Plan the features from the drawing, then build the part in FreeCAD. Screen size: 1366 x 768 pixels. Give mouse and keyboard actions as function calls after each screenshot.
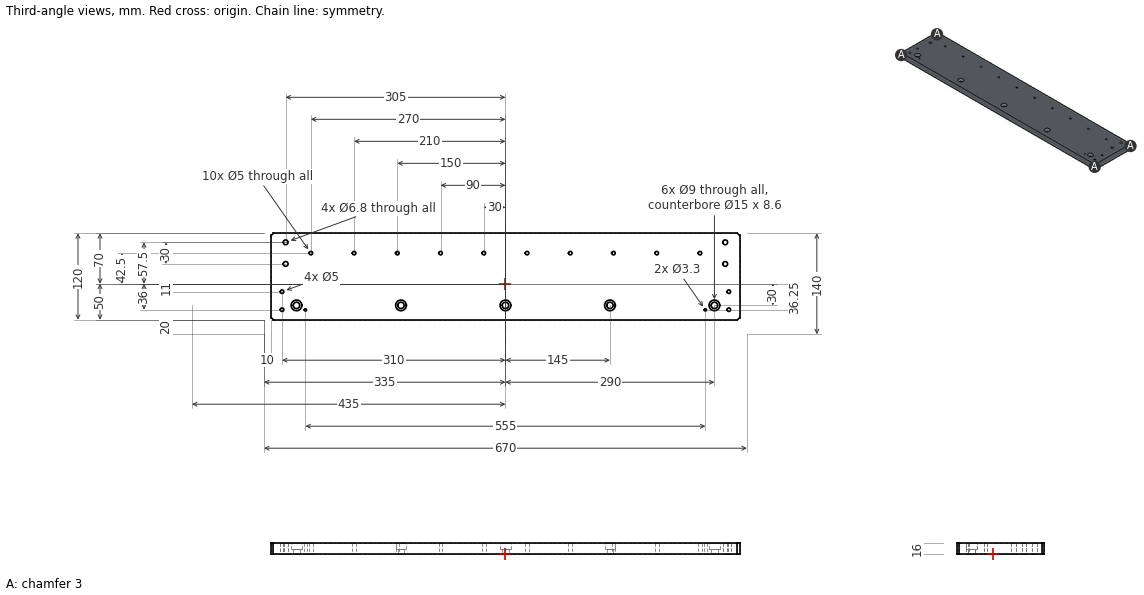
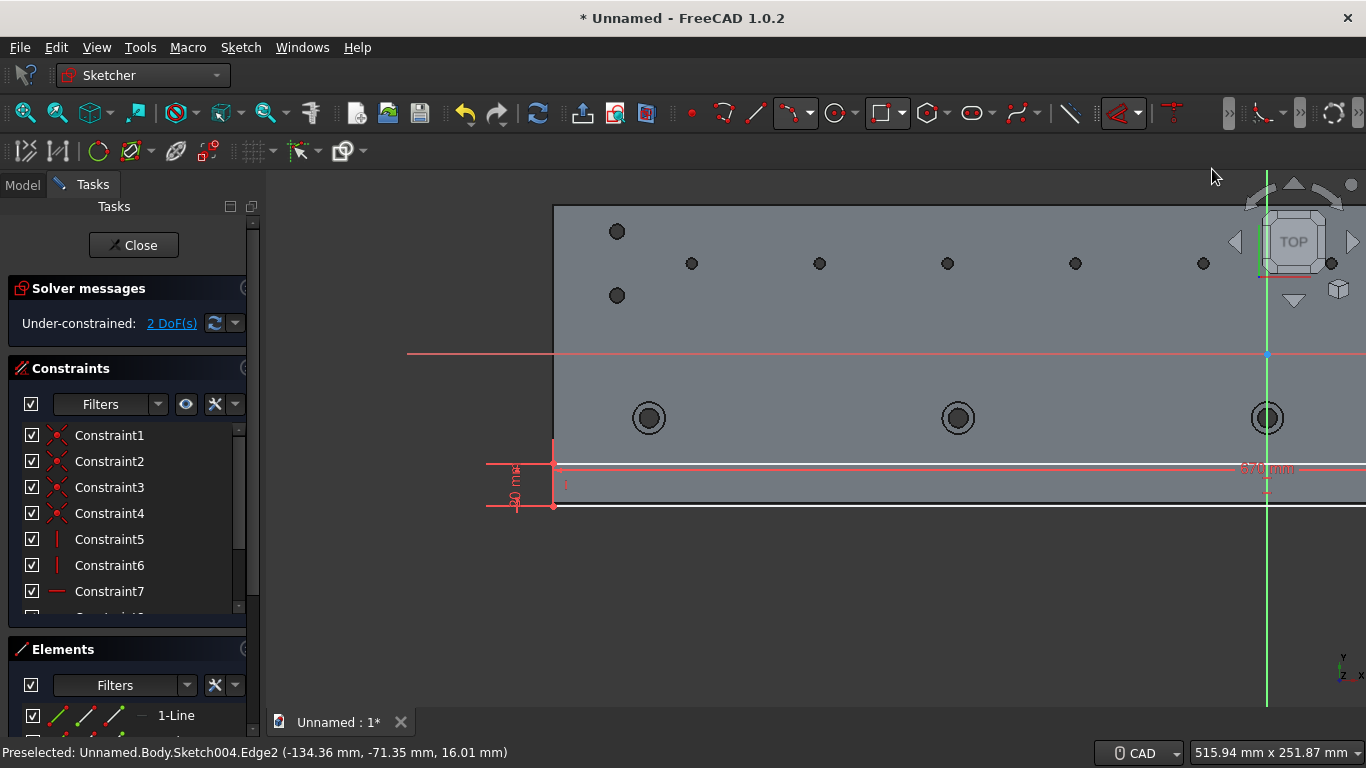
click(553, 464)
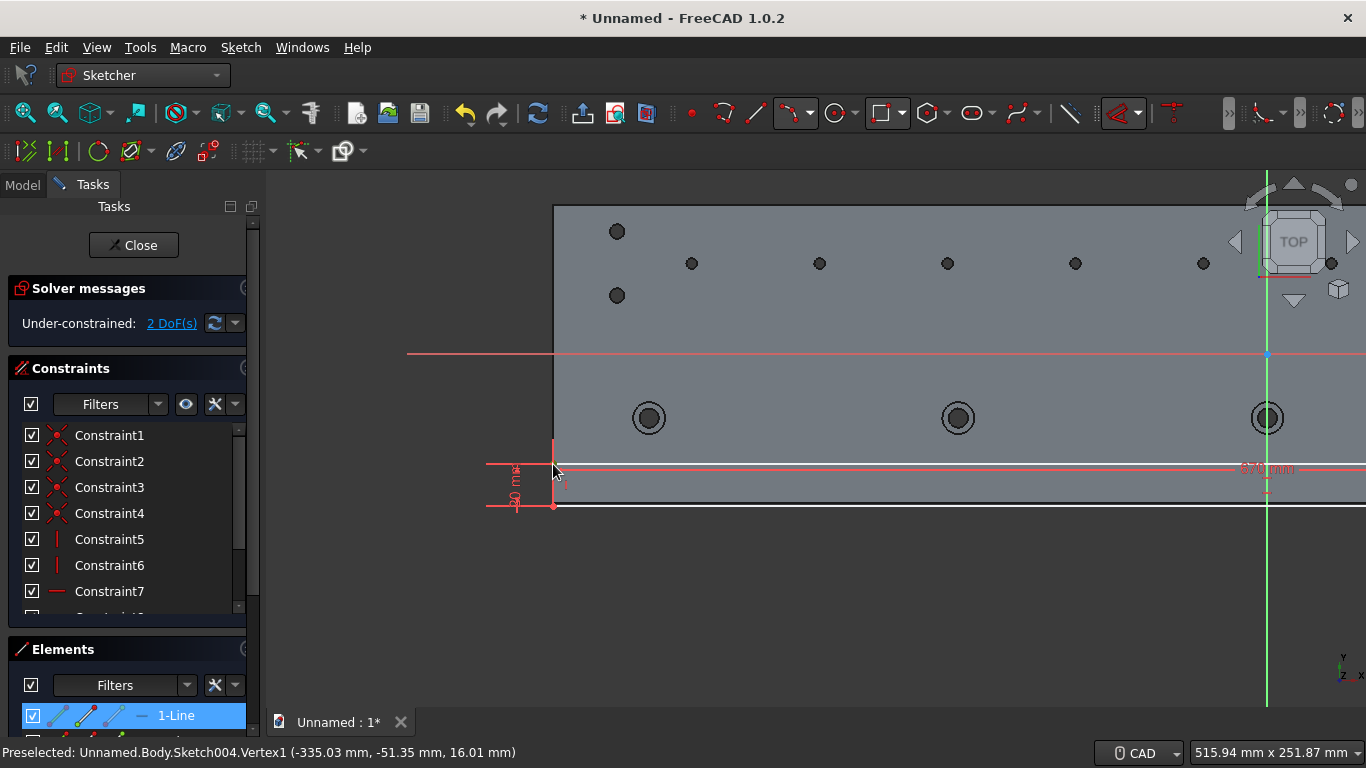
key(i)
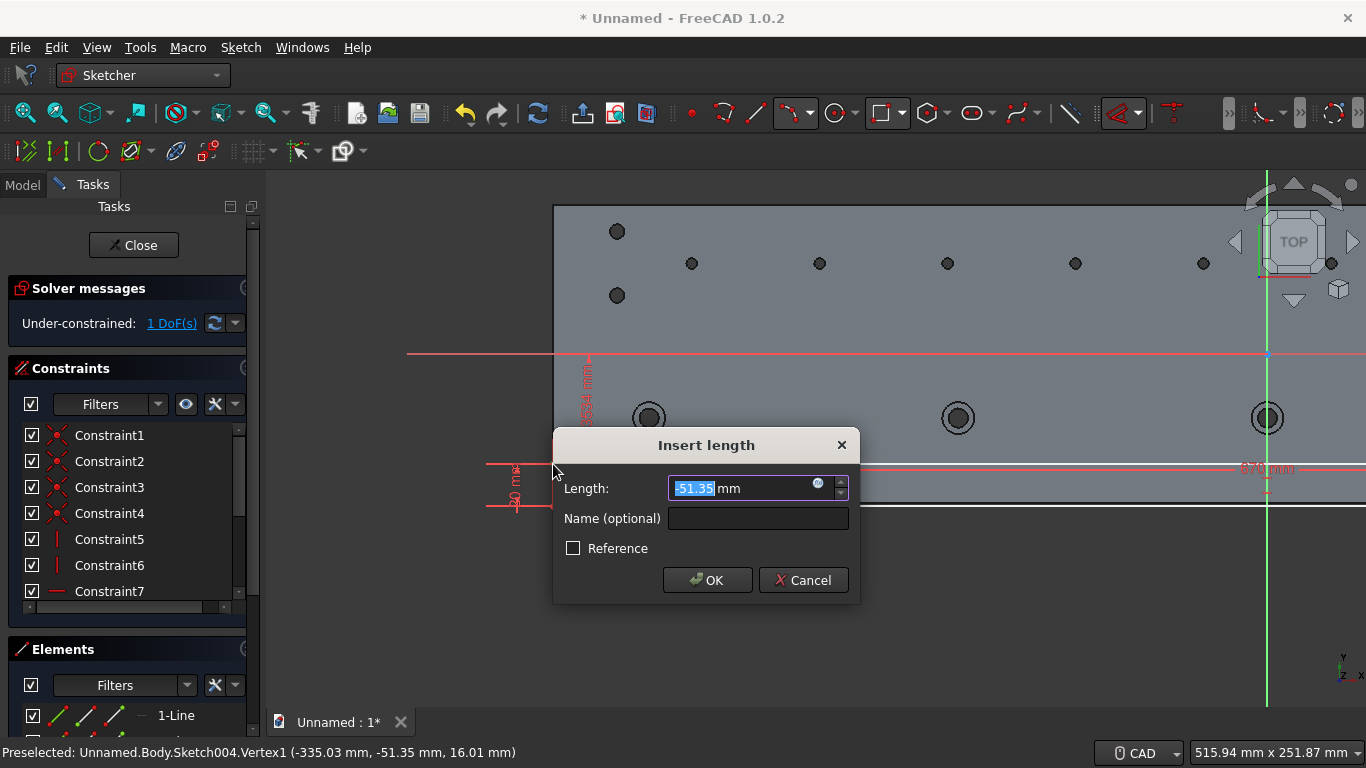
text(-50)
key(Return)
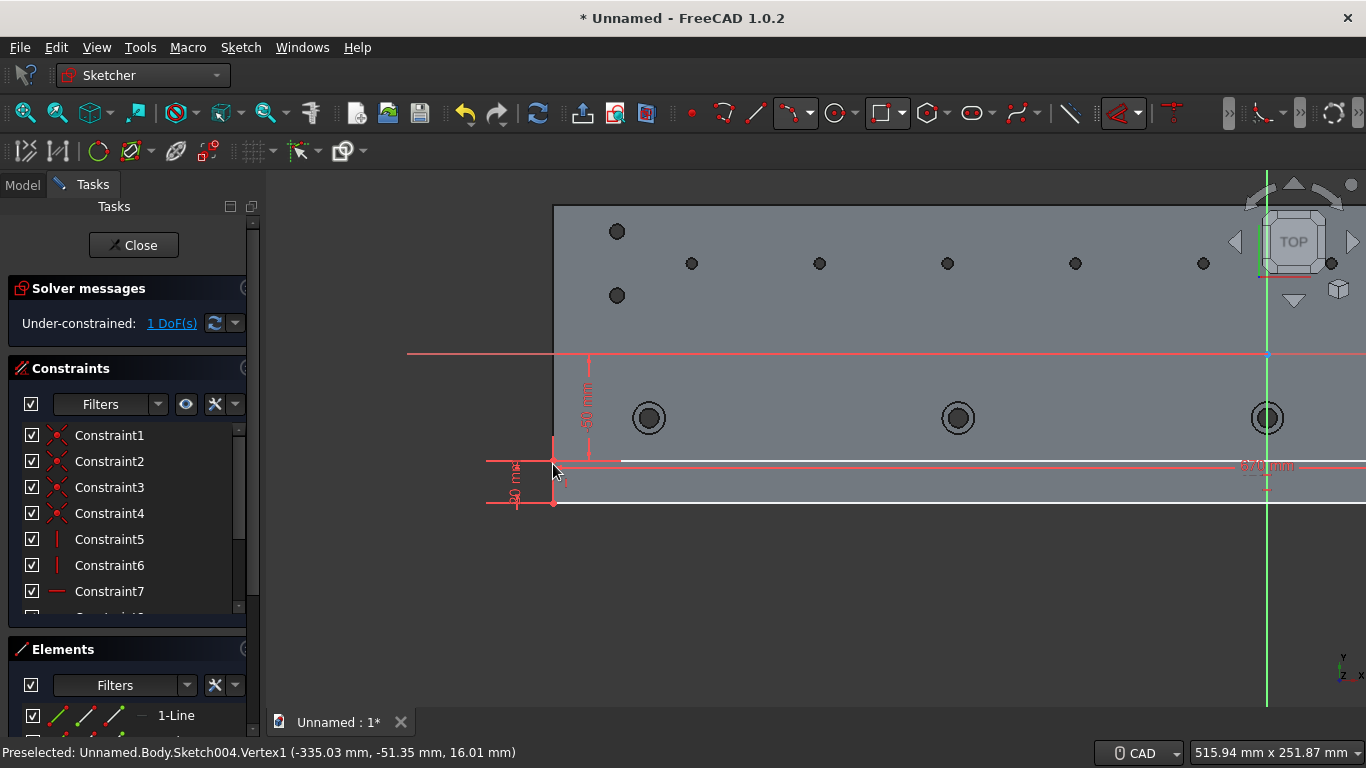
click(553, 461)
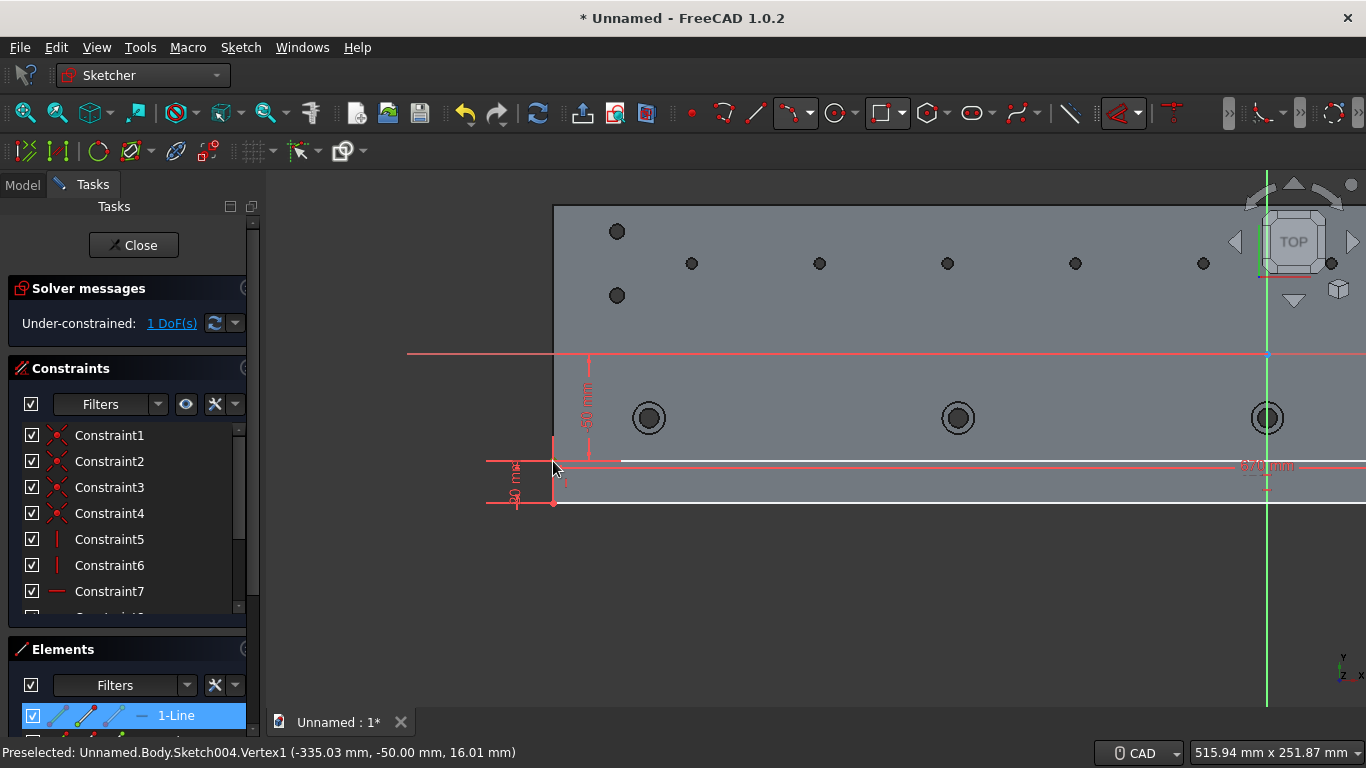
click(1140, 114)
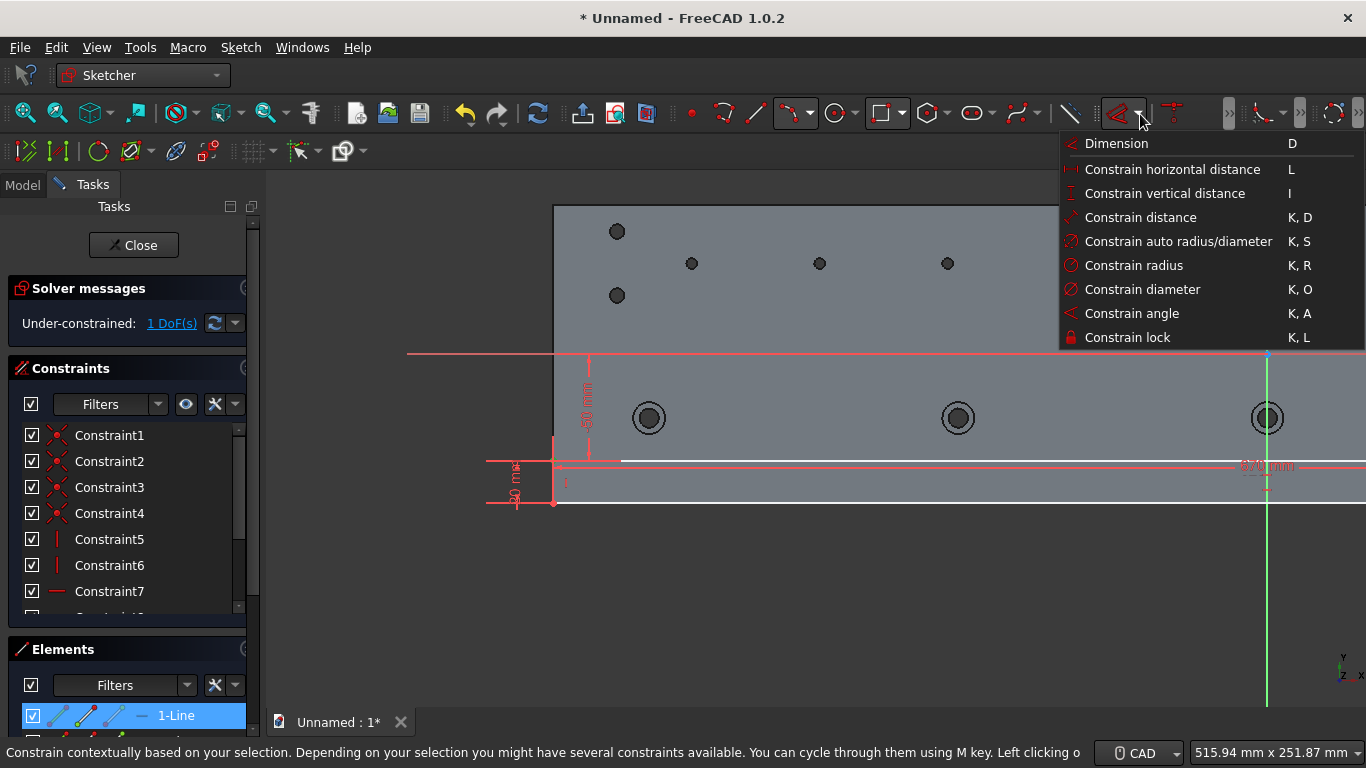
click(1212, 169)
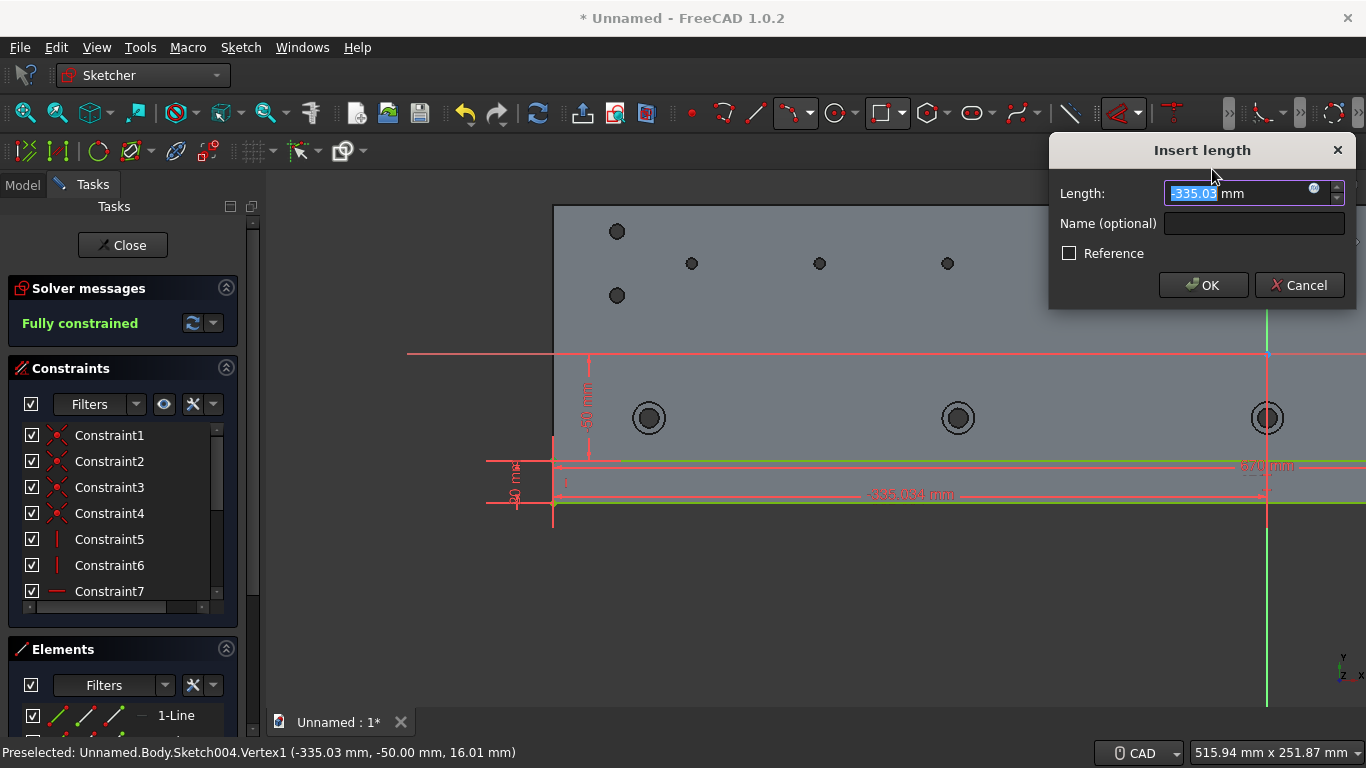
text(-335)
key(Return)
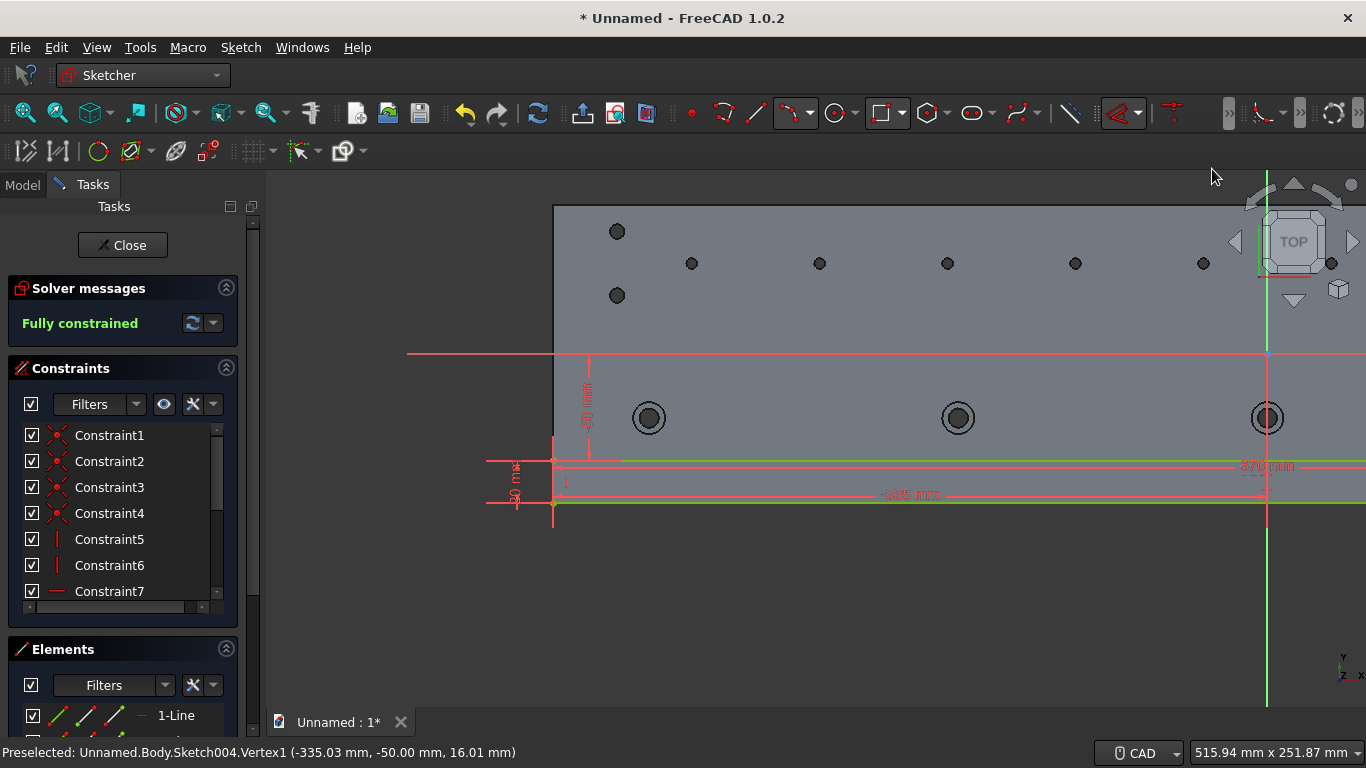
click(123, 245)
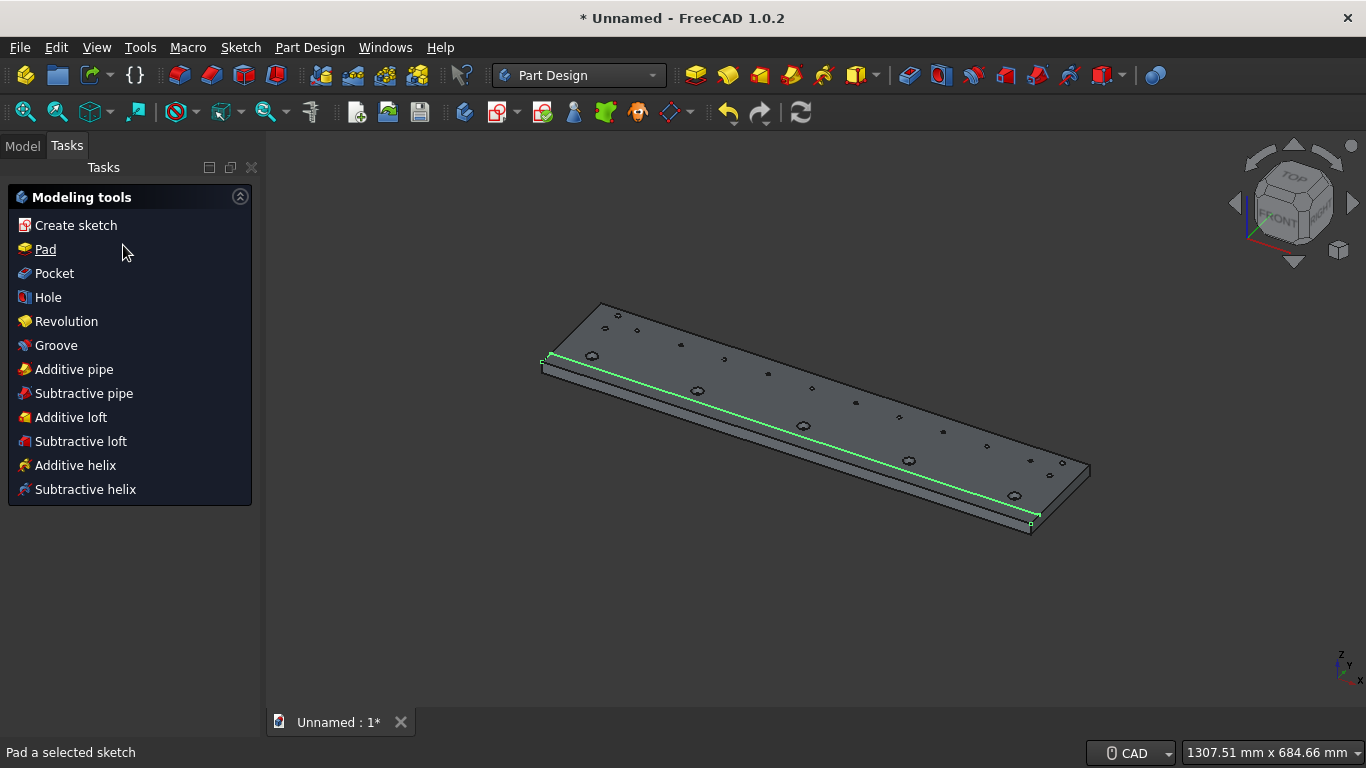
click(910, 76)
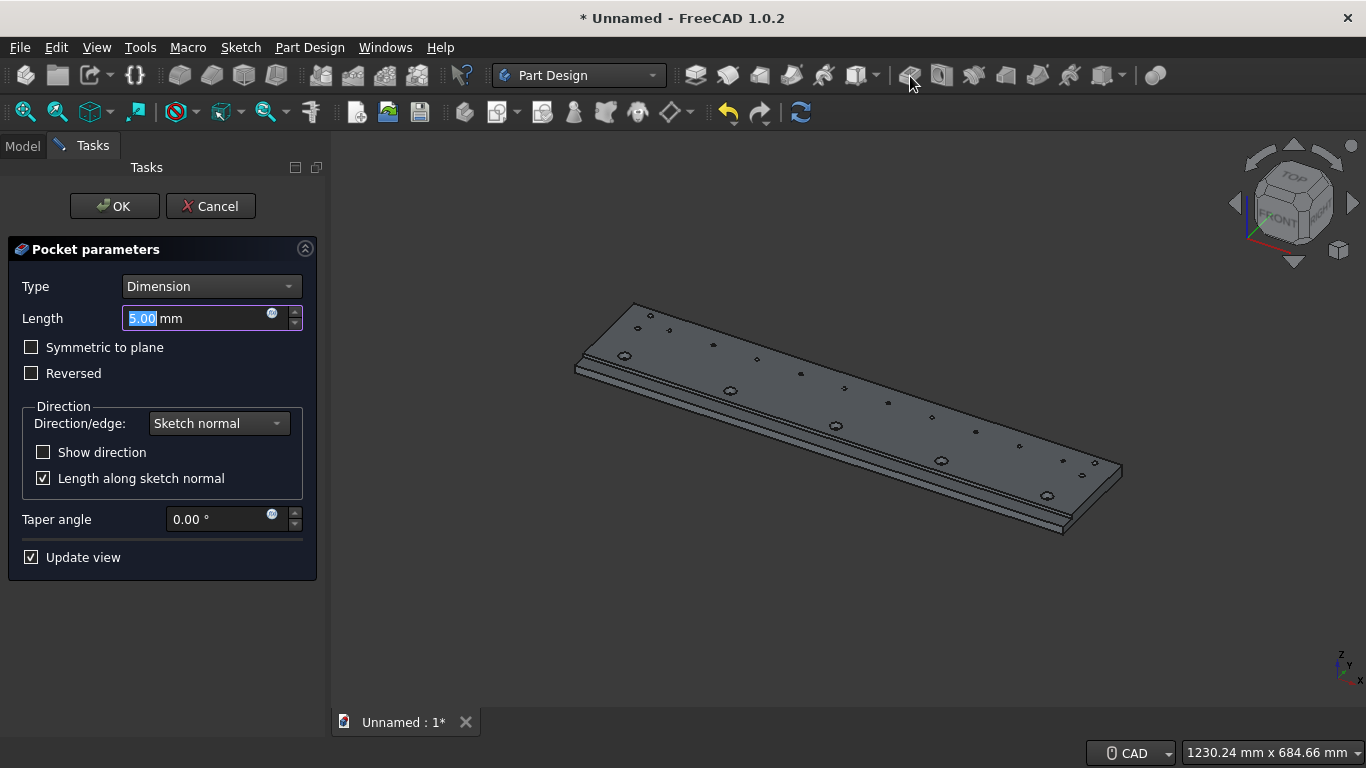
click(212, 286)